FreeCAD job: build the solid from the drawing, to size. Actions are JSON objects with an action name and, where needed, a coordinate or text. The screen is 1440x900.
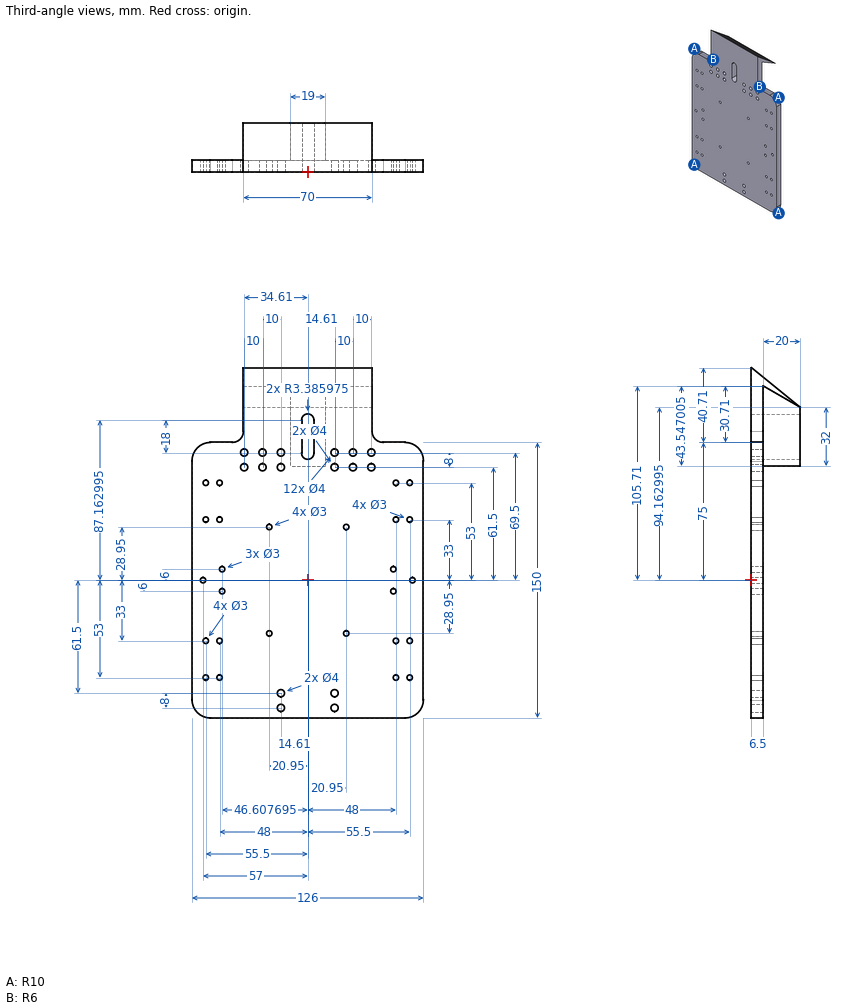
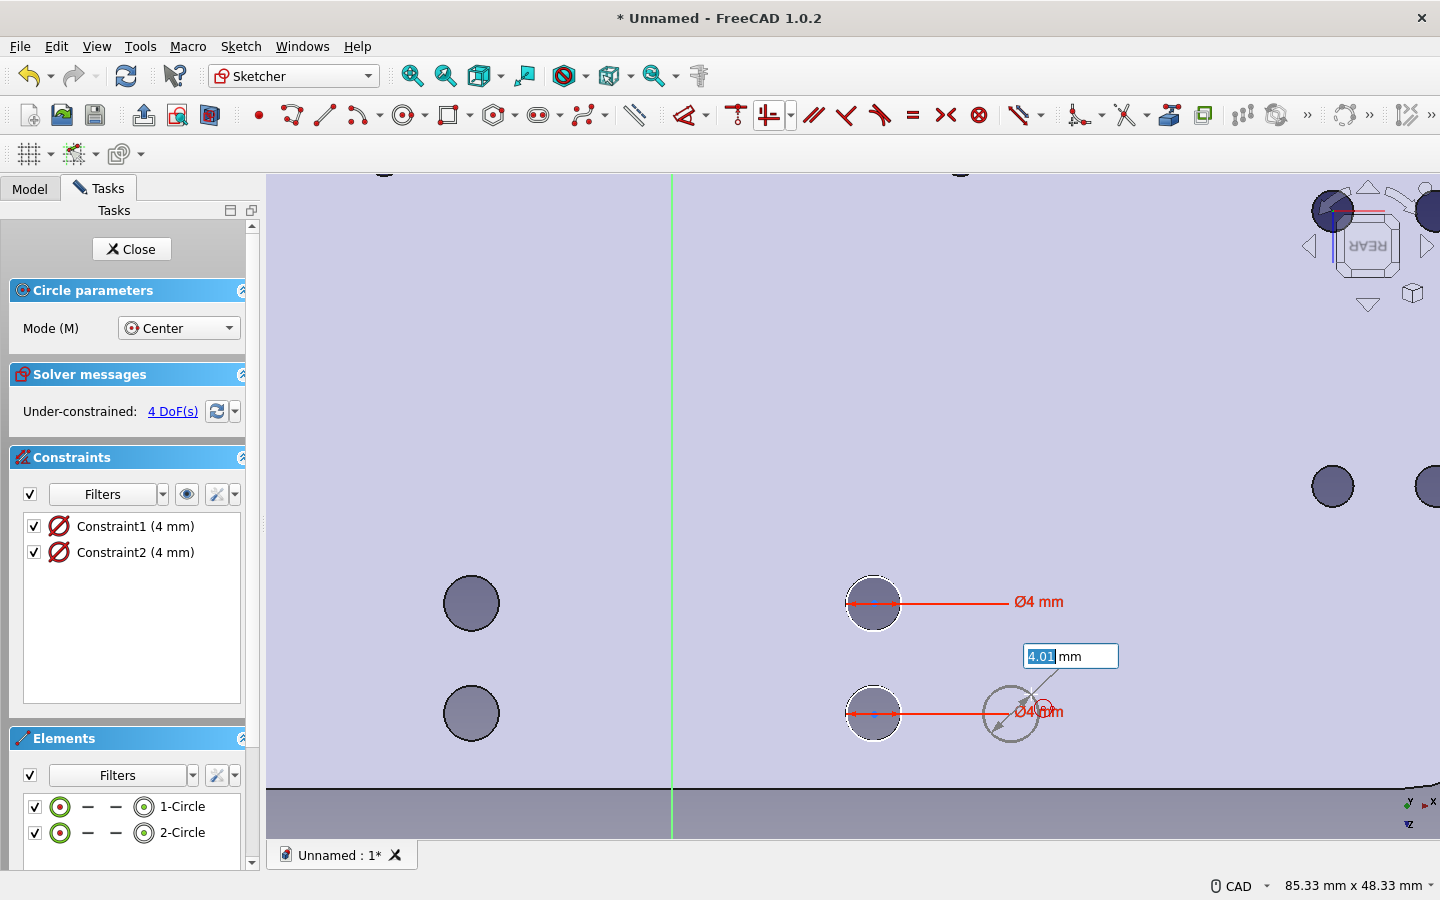
{"action": "type", "text": "4"}
{"action": "key", "text": "Return"}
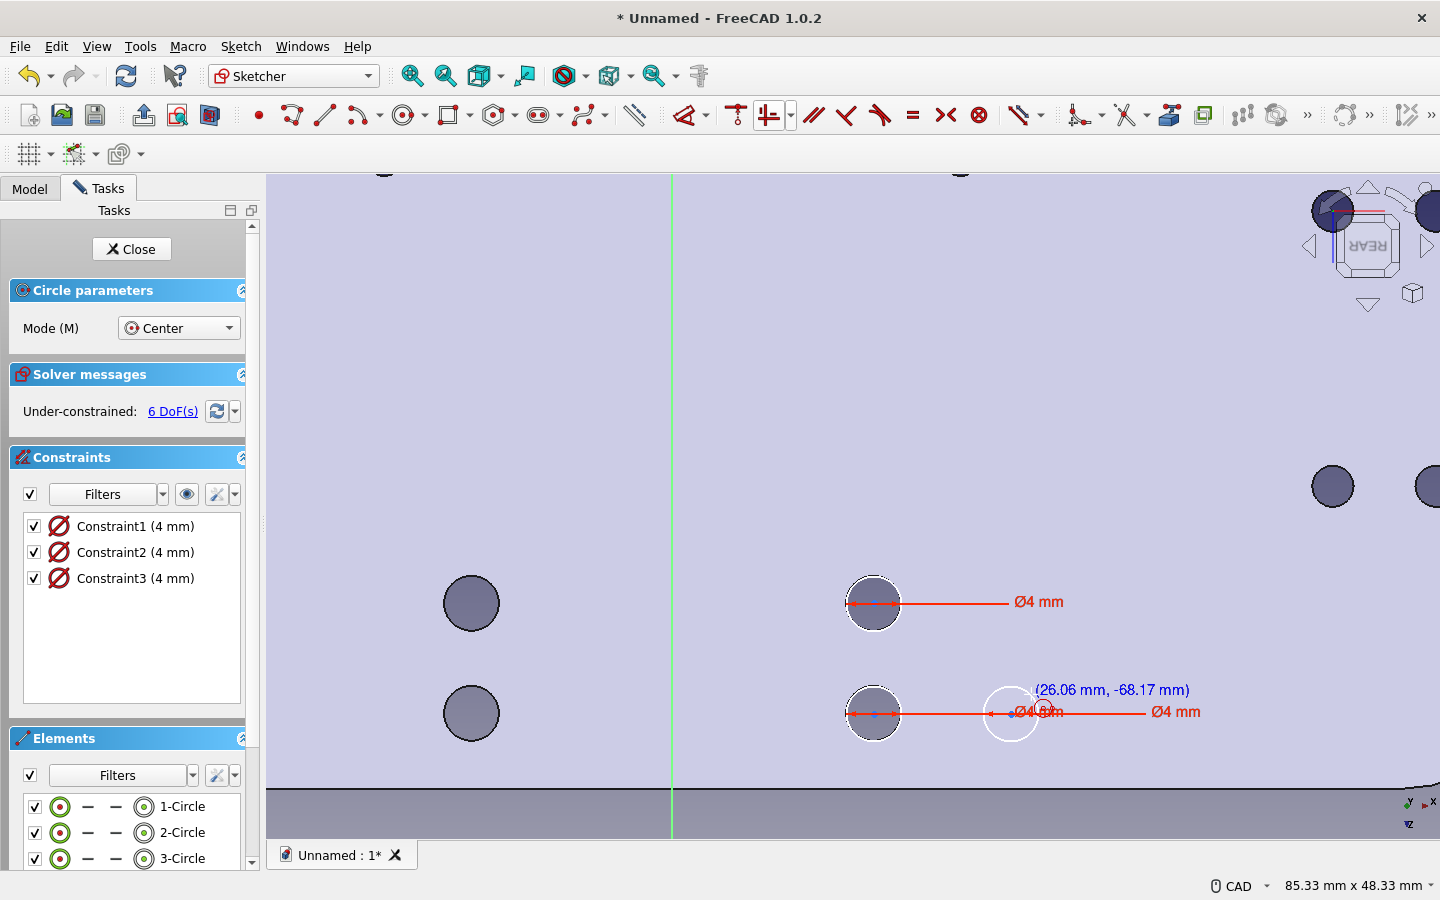
{"action": "left_click", "coordinate": [1011, 603]}
{"action": "mouse_move", "coordinate": [1031, 584]}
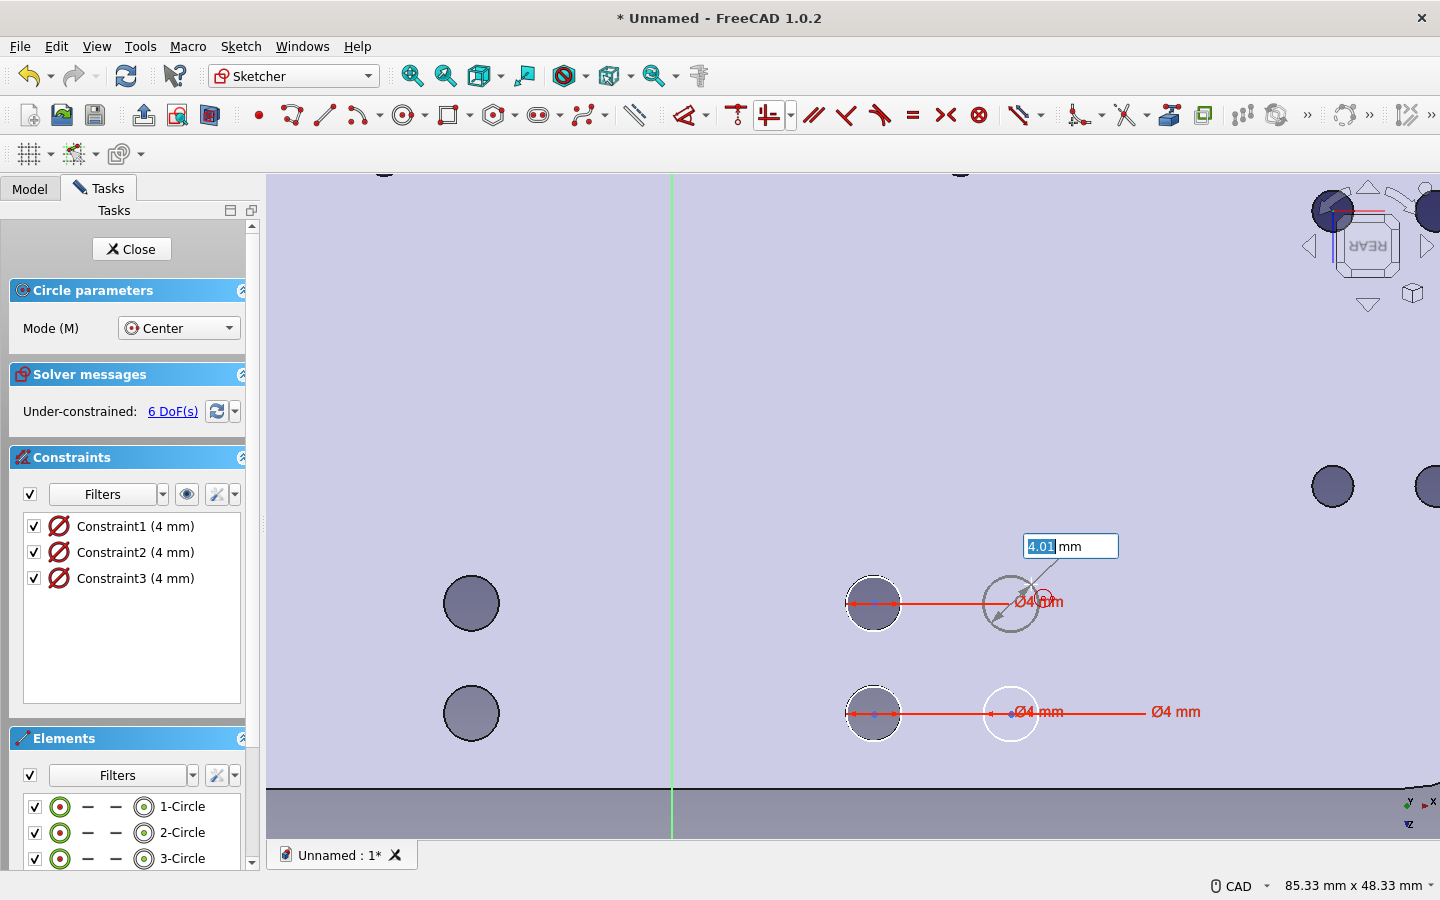
{"action": "type", "text": "4"}
{"action": "key", "text": "Return"}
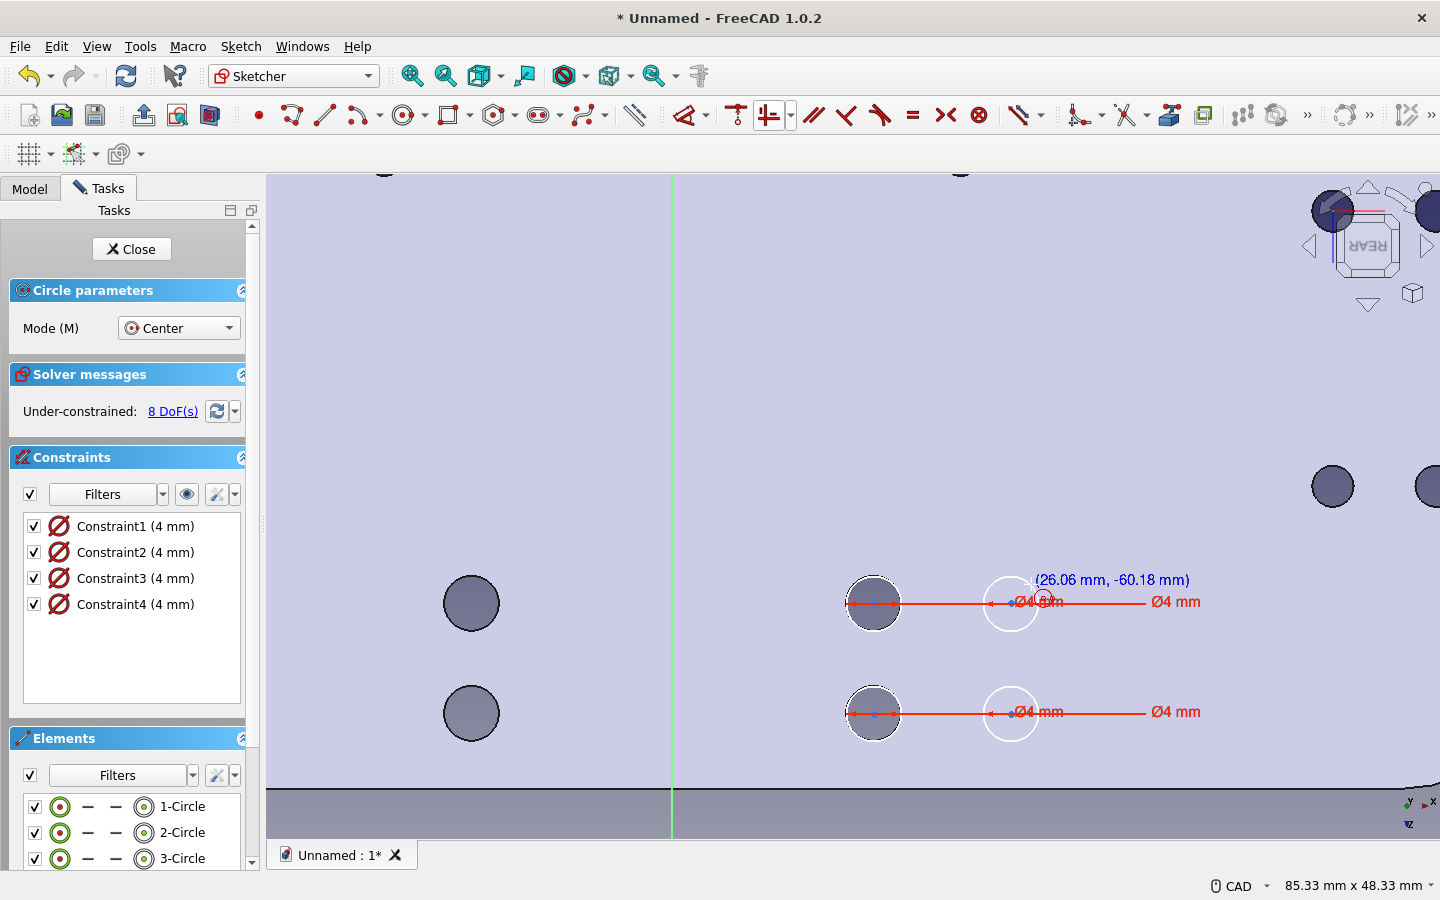
{"action": "left_click", "coordinate": [1149, 713]}
{"action": "mouse_move", "coordinate": [1168, 694]}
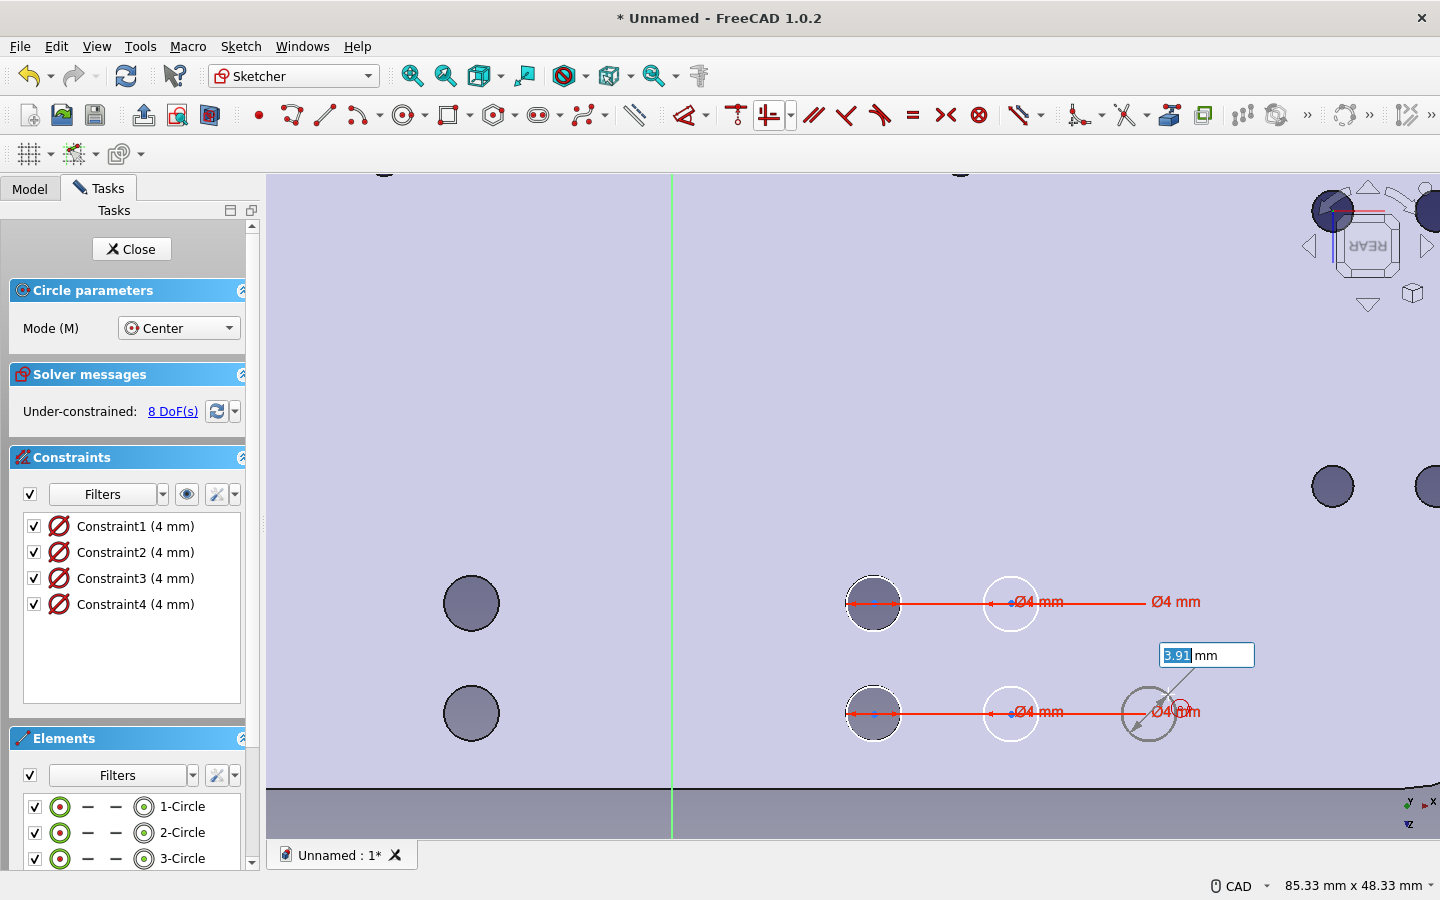
{"action": "type", "text": "4"}
{"action": "key", "text": "Return"}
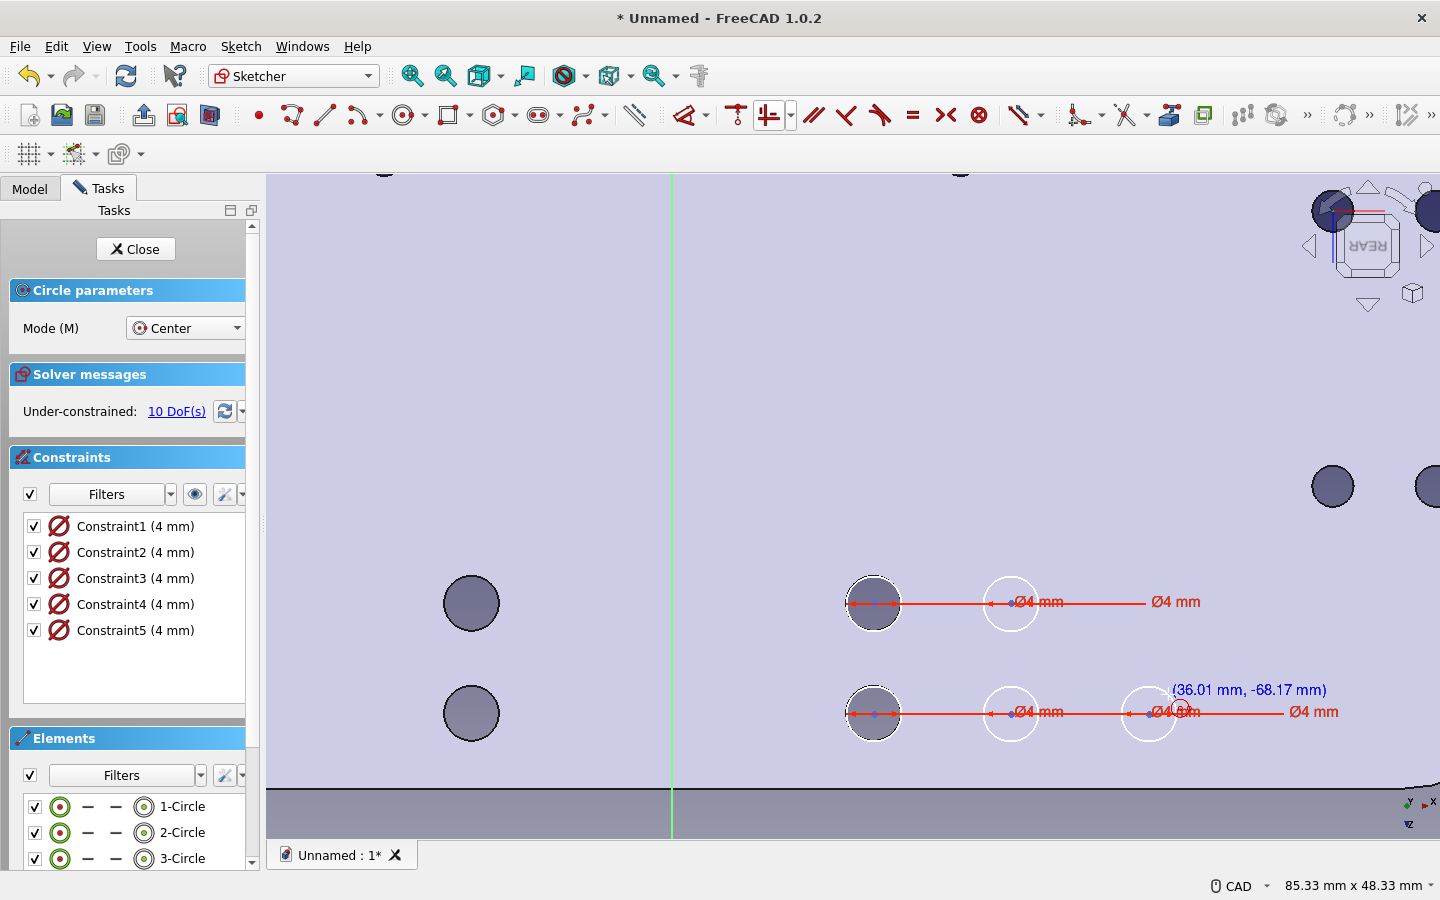
{"action": "left_click", "coordinate": [1149, 603]}
{"action": "mouse_move", "coordinate": [1168, 584]}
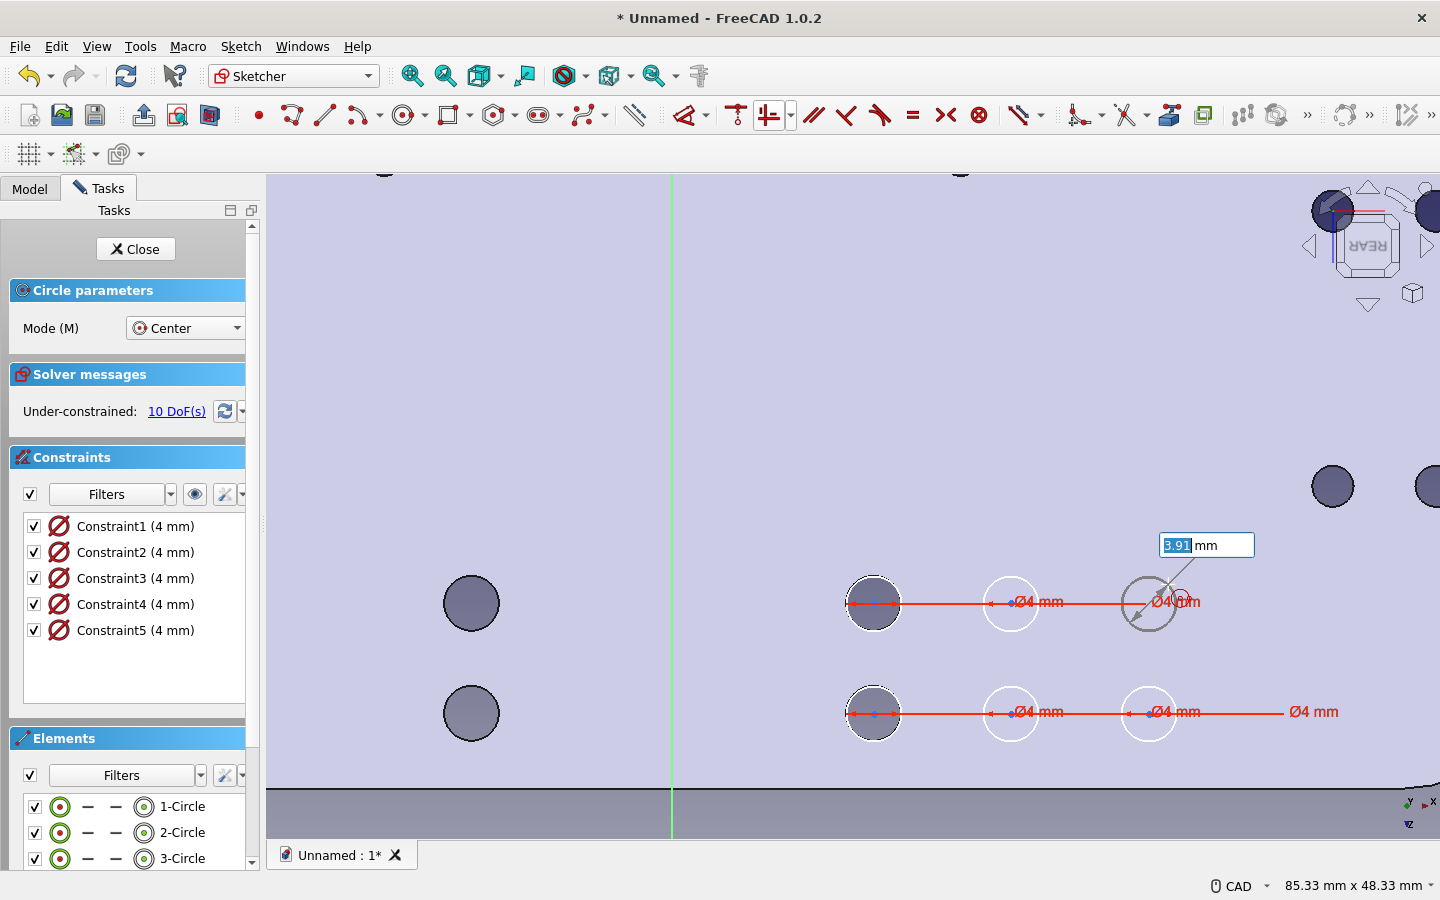
{"action": "type", "text": "4"}
{"action": "key", "text": "Return"}